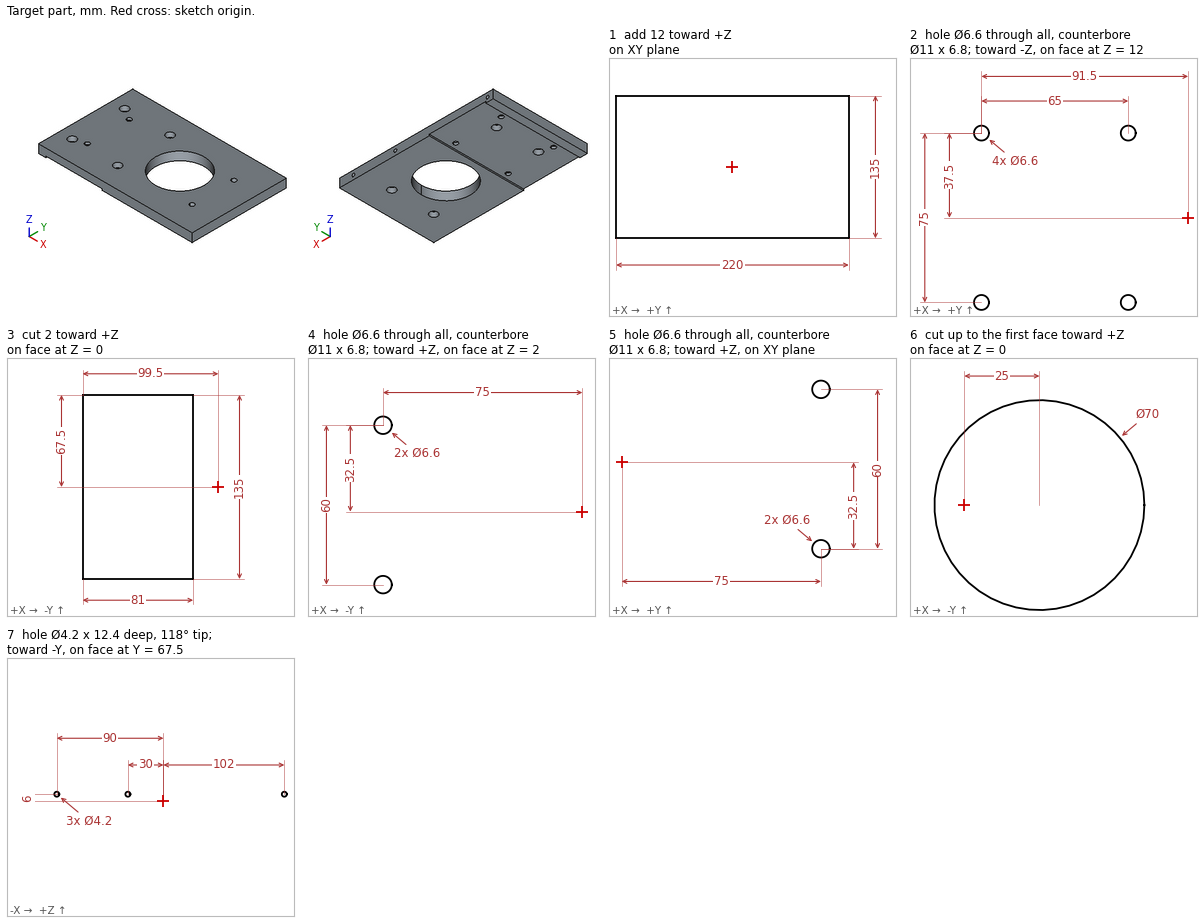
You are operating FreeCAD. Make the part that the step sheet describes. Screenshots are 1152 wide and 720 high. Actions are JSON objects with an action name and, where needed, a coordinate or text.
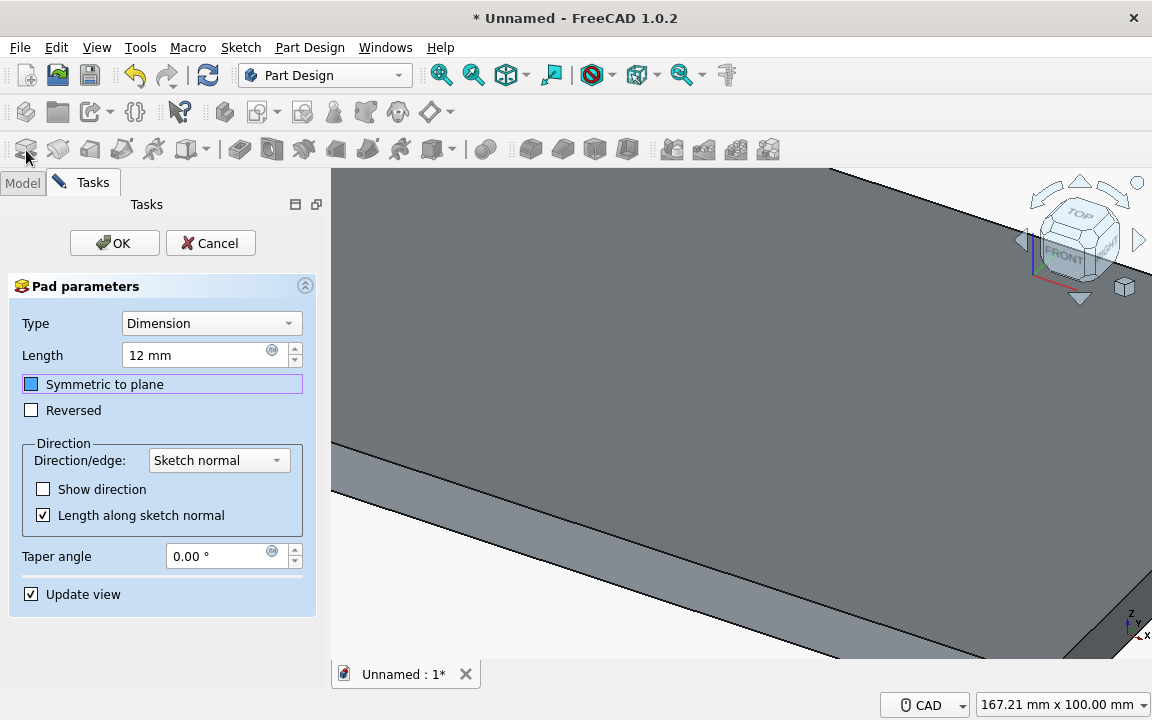
{"action": "left_click", "coordinate": [115, 243]}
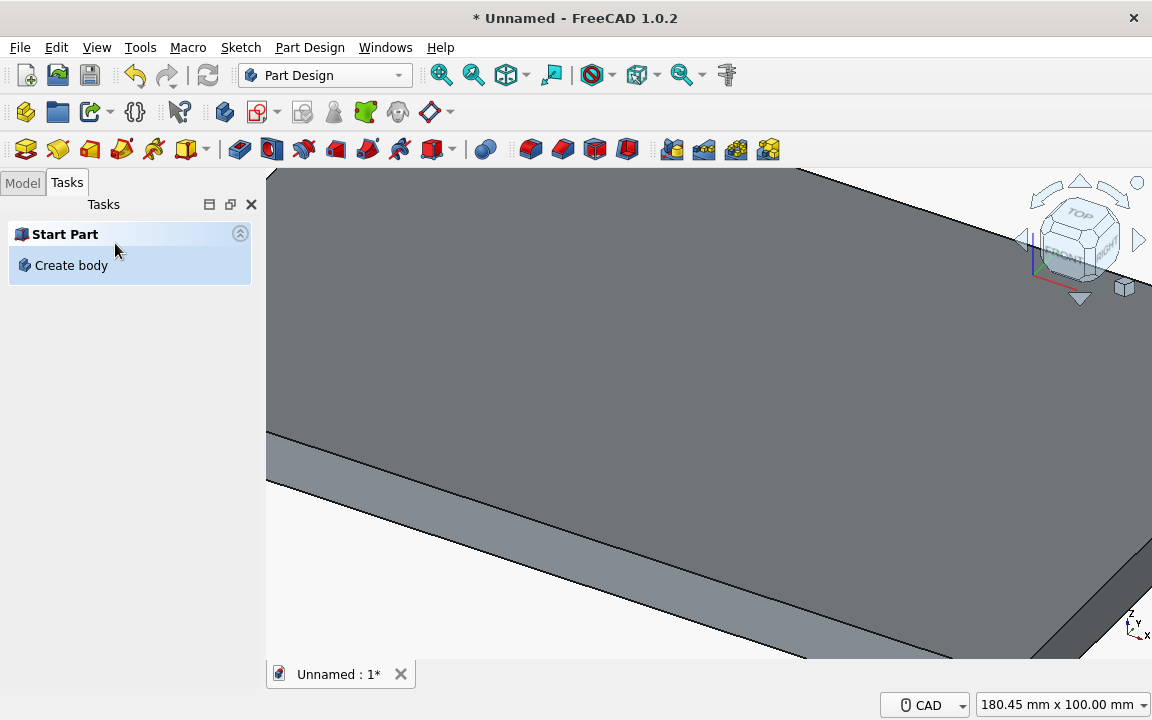
{"action": "key", "text": "v f"}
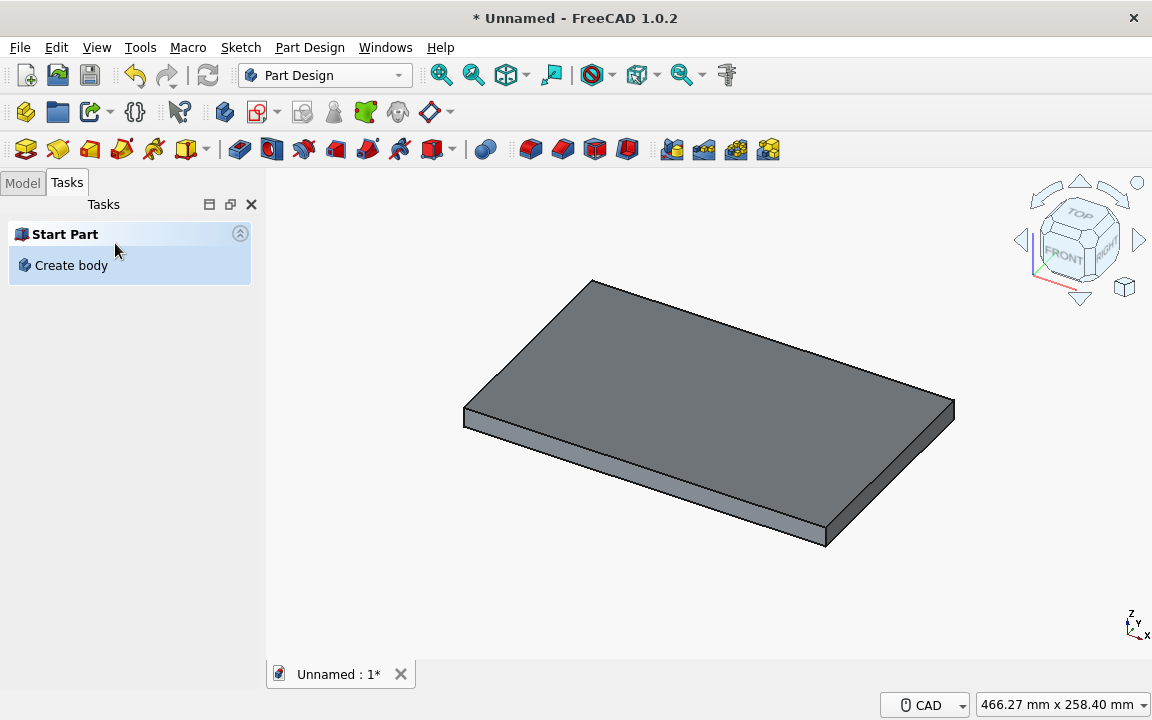
{"action": "left_click", "coordinate": [761, 420]}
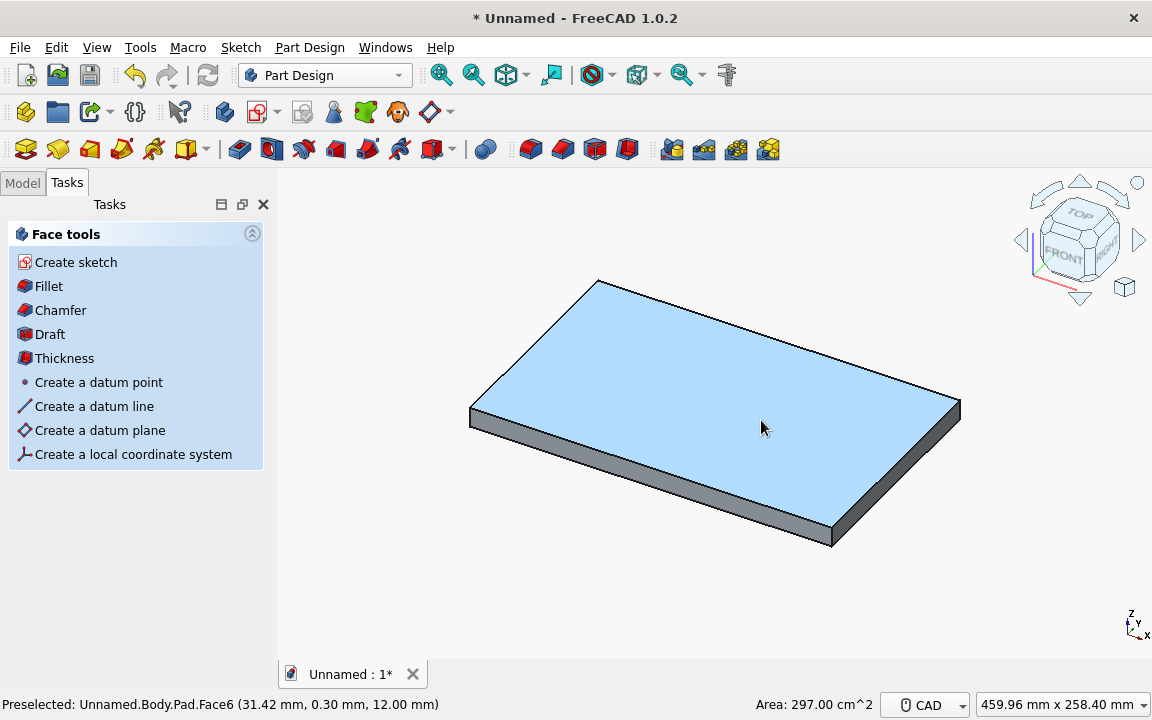
{"action": "left_click", "coordinate": [258, 112]}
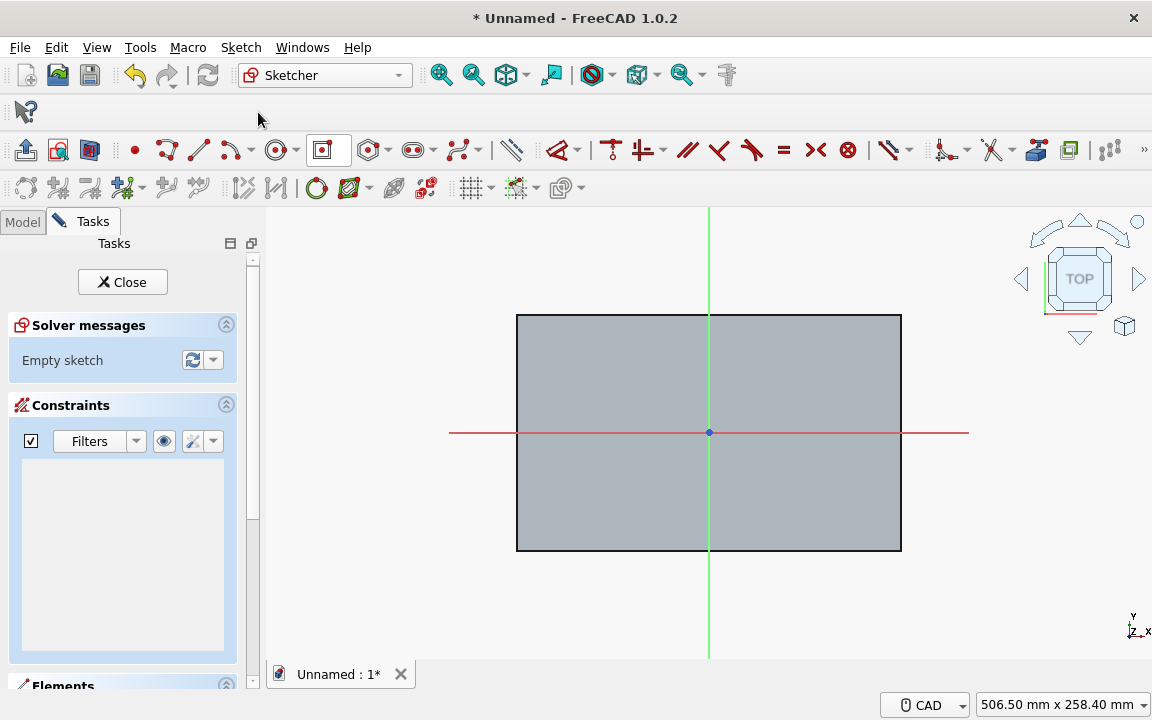
{"action": "scroll", "coordinate": [609, 433], "scroll_direction": "up", "scroll_amount": 3}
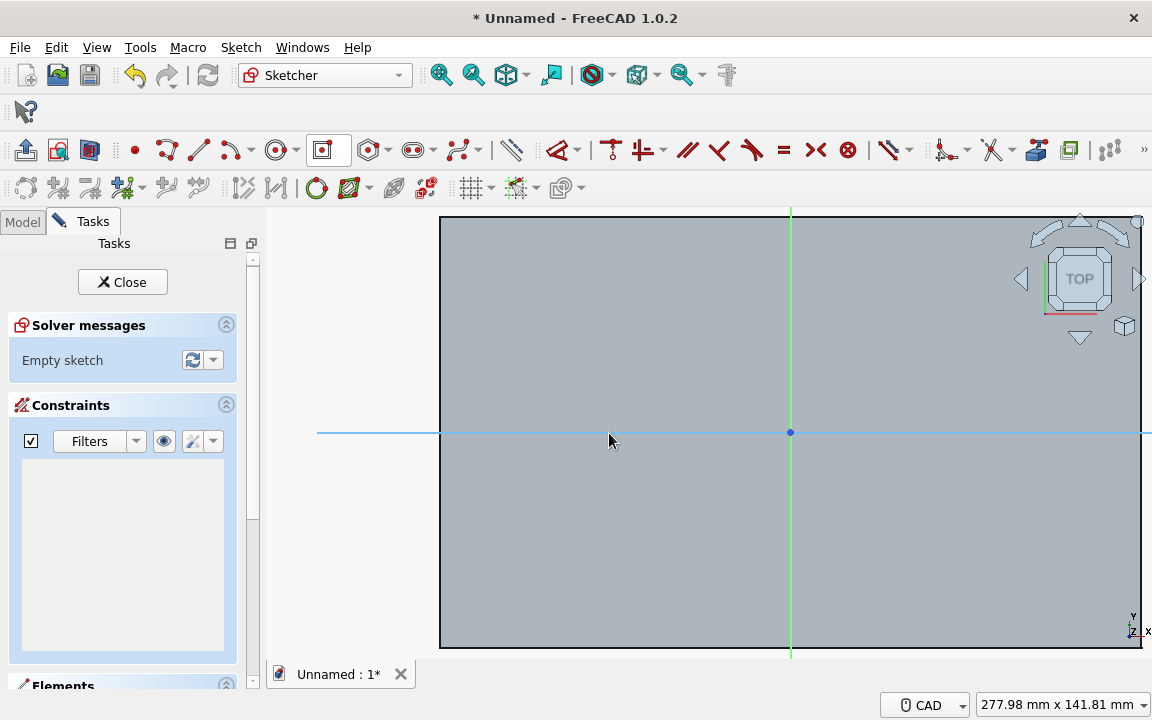
{"action": "key", "text": "g c"}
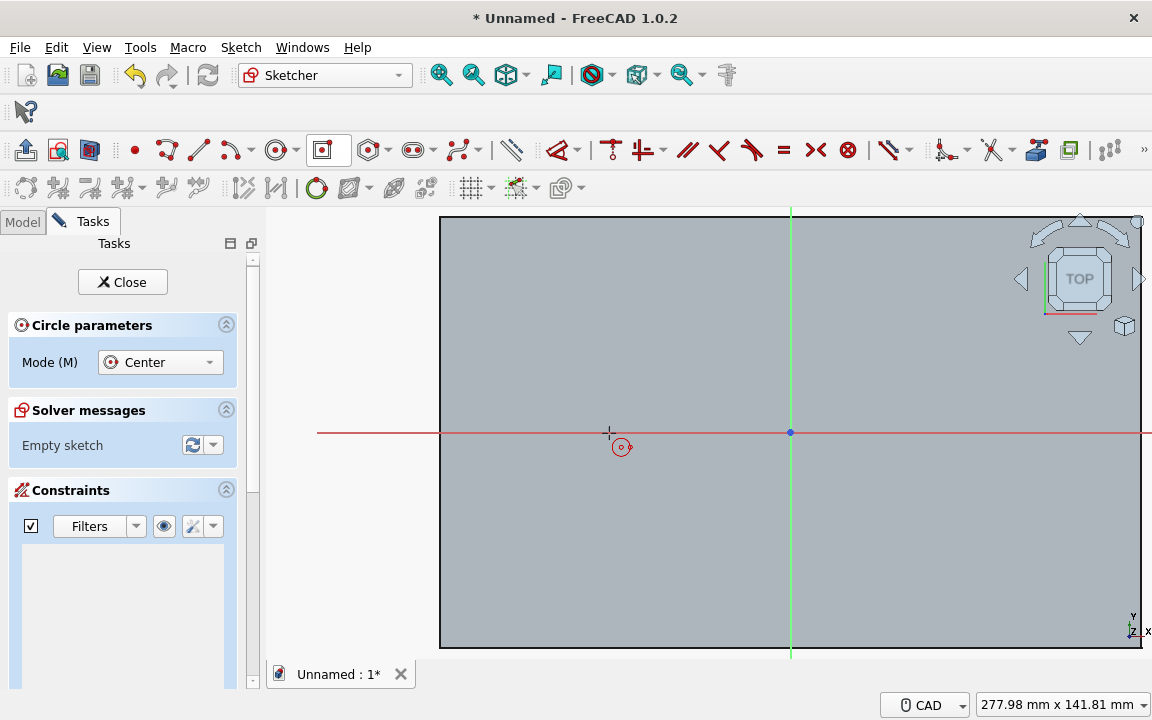
{"action": "scroll", "coordinate": [499, 313], "scroll_direction": "up", "scroll_amount": 4}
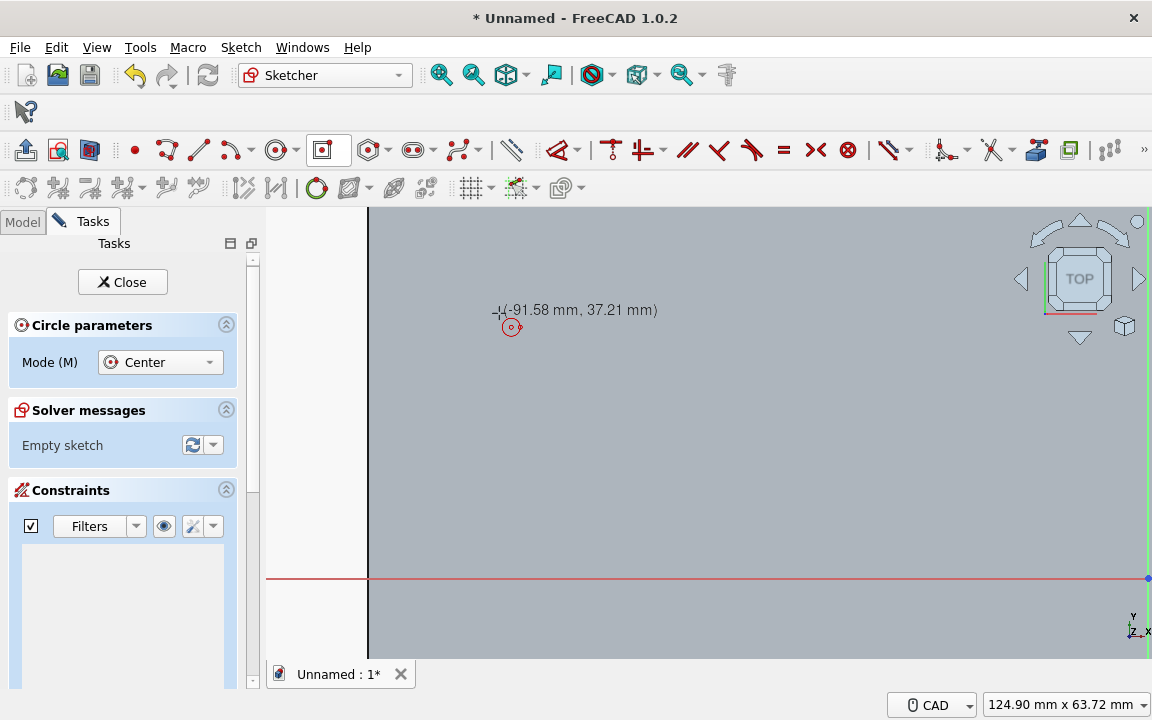
{"action": "left_click", "coordinate": [499, 313]}
{"action": "mouse_move", "coordinate": [516, 296]}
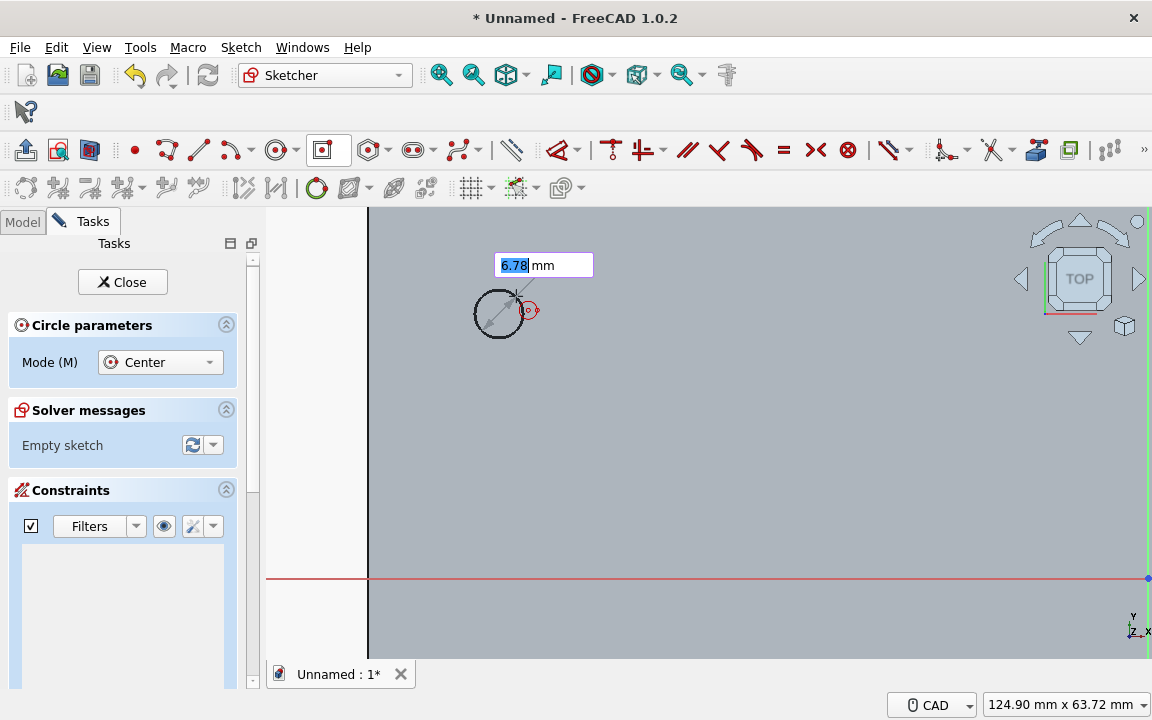
{"action": "type", "text": "6.6"}
{"action": "key", "text": "Return"}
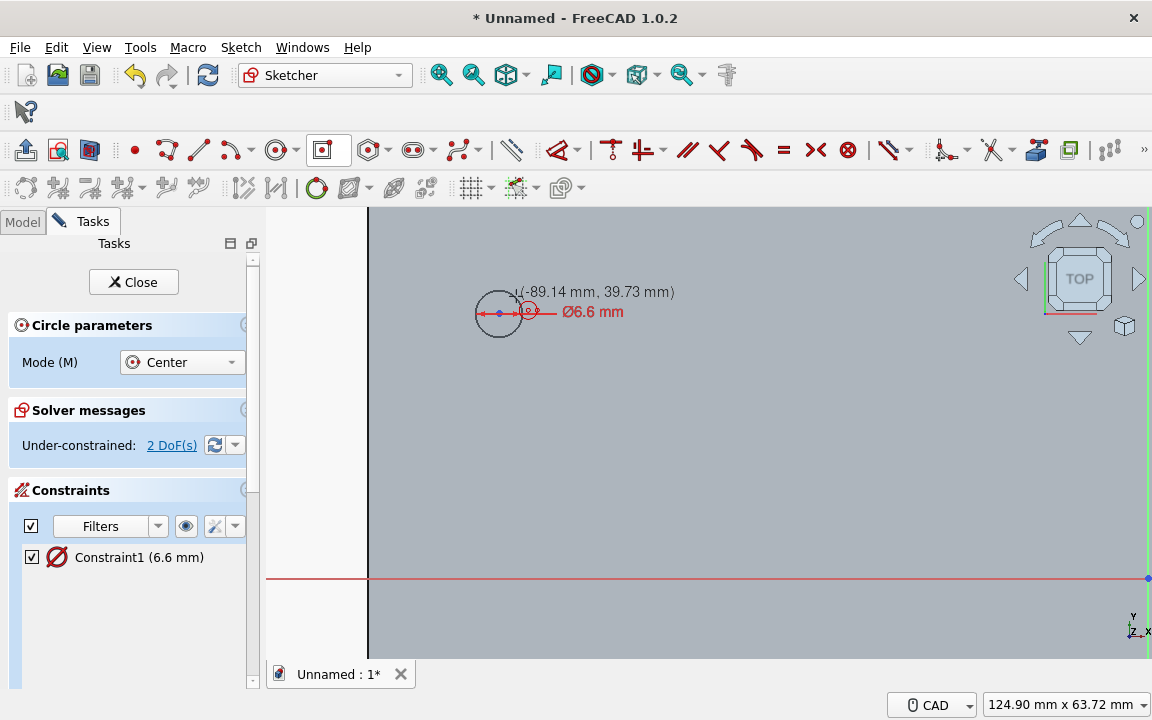
{"action": "left_click", "coordinate": [960, 313]}
{"action": "mouse_move", "coordinate": [977, 296]}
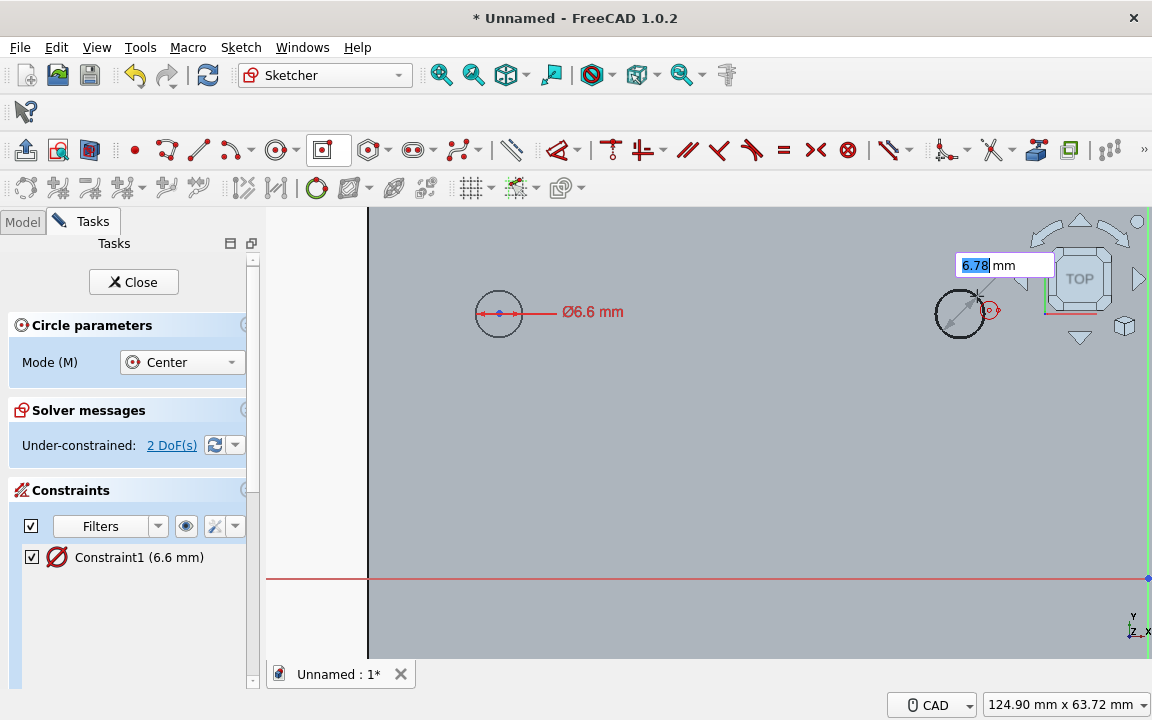
{"action": "type", "text": "6.6"}
{"action": "key", "text": "Return"}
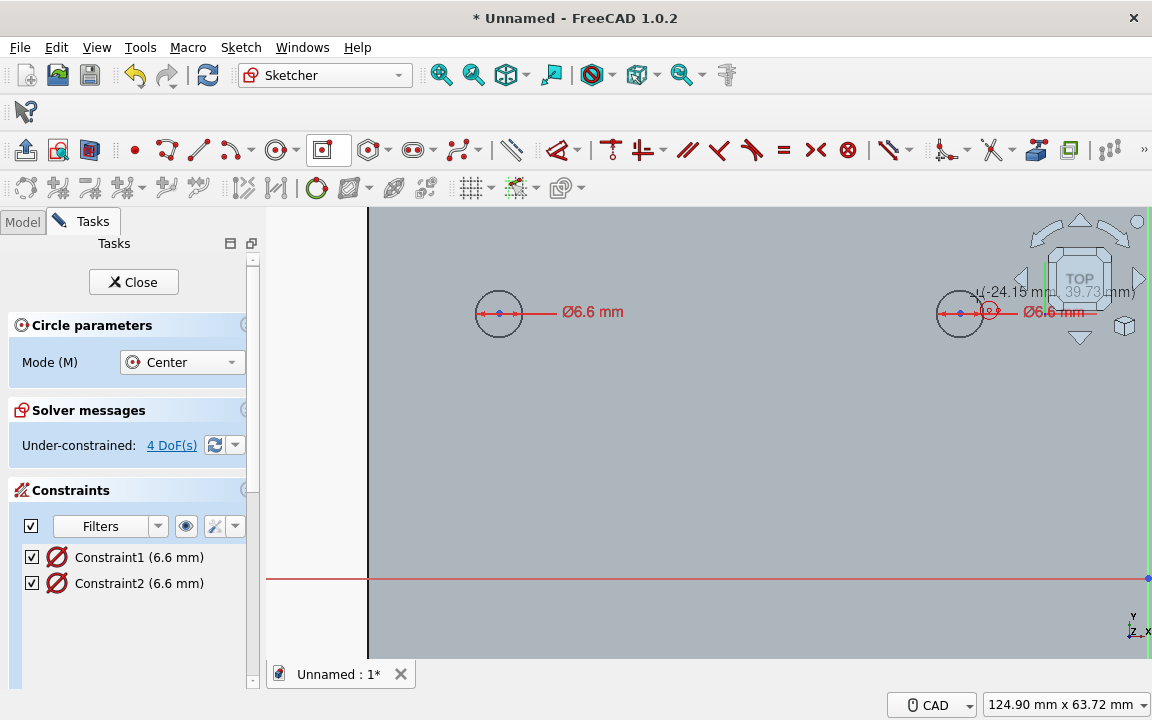
{"action": "scroll", "coordinate": [501, 314], "scroll_direction": "down", "scroll_amount": 4}